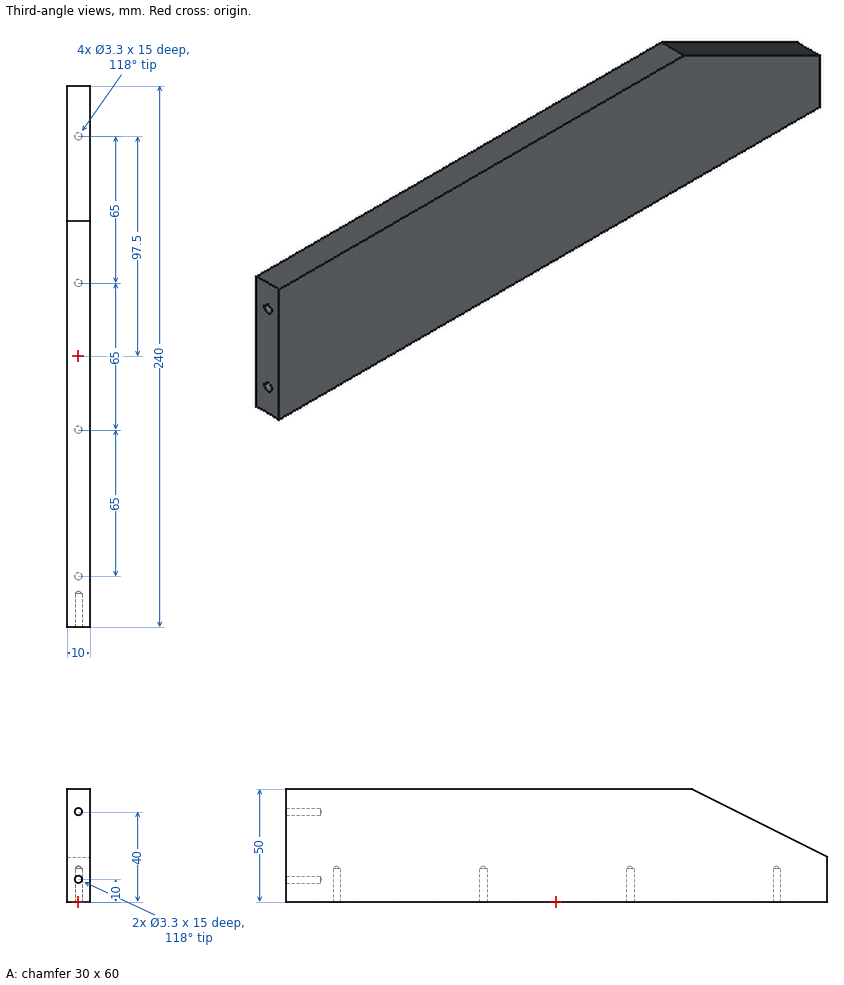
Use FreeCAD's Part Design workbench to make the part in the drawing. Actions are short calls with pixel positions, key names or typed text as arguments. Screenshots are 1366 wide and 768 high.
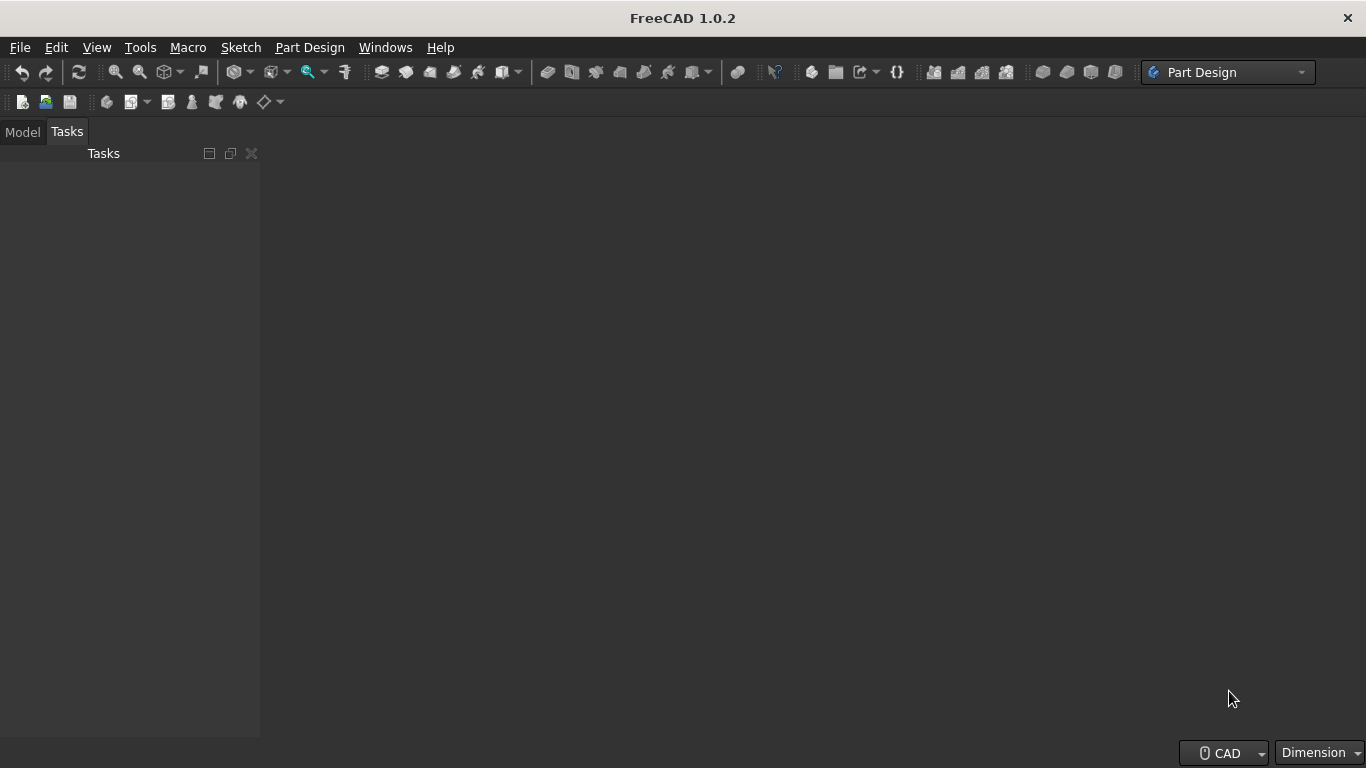
click(22, 102)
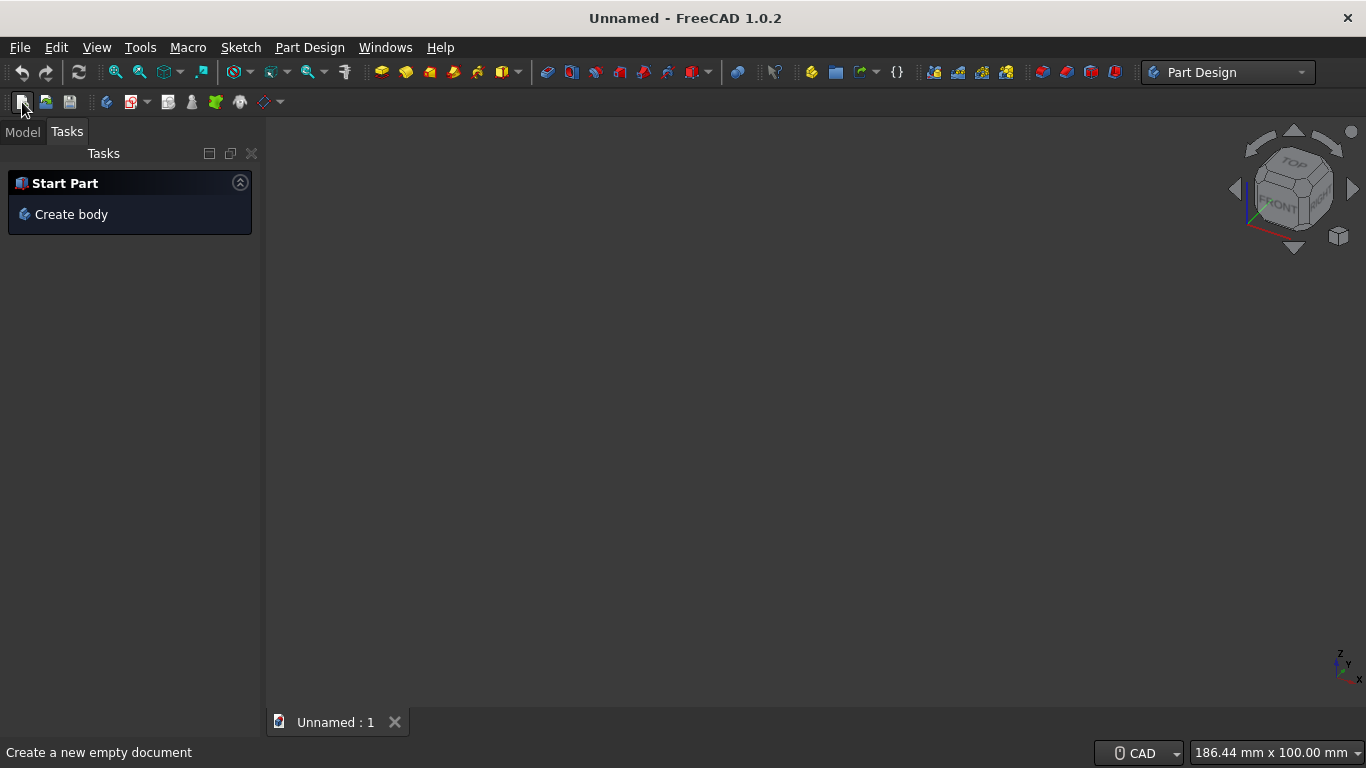
click(132, 102)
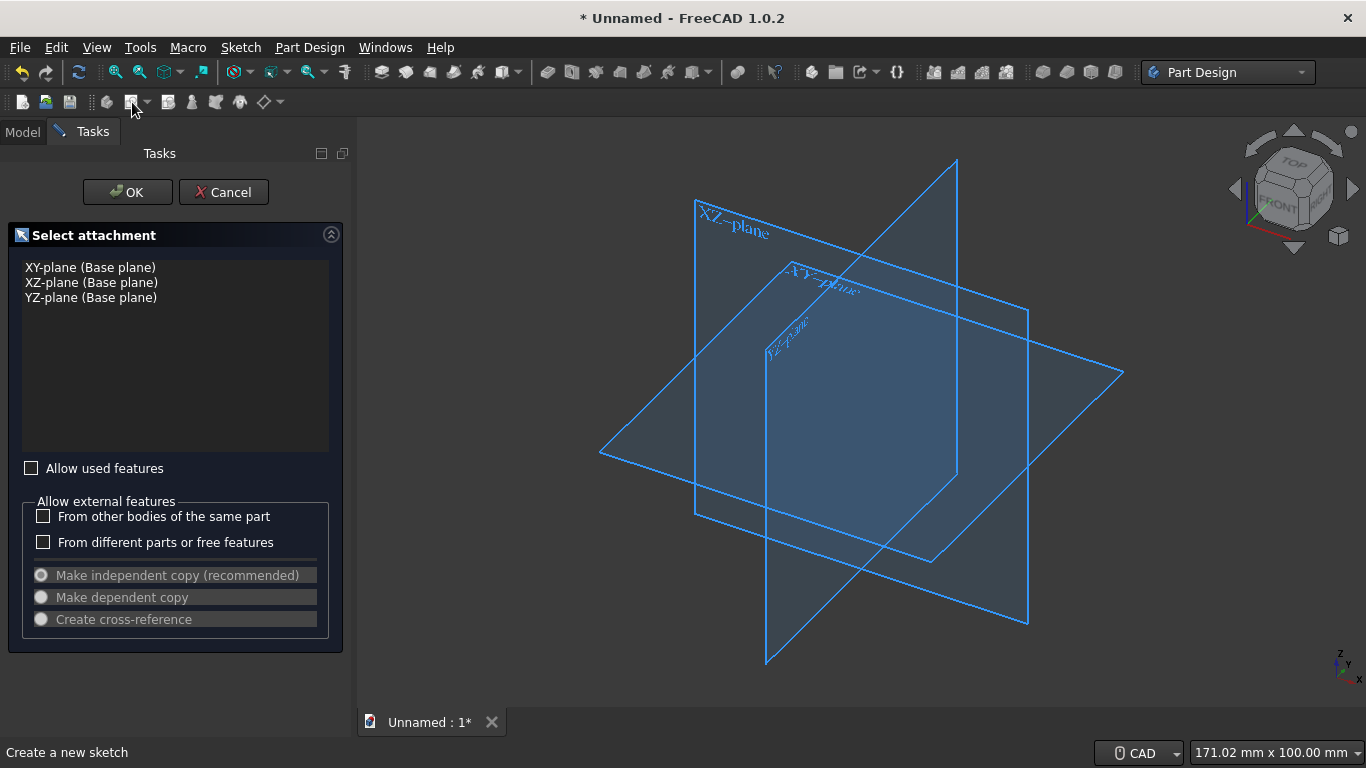
click(82, 268)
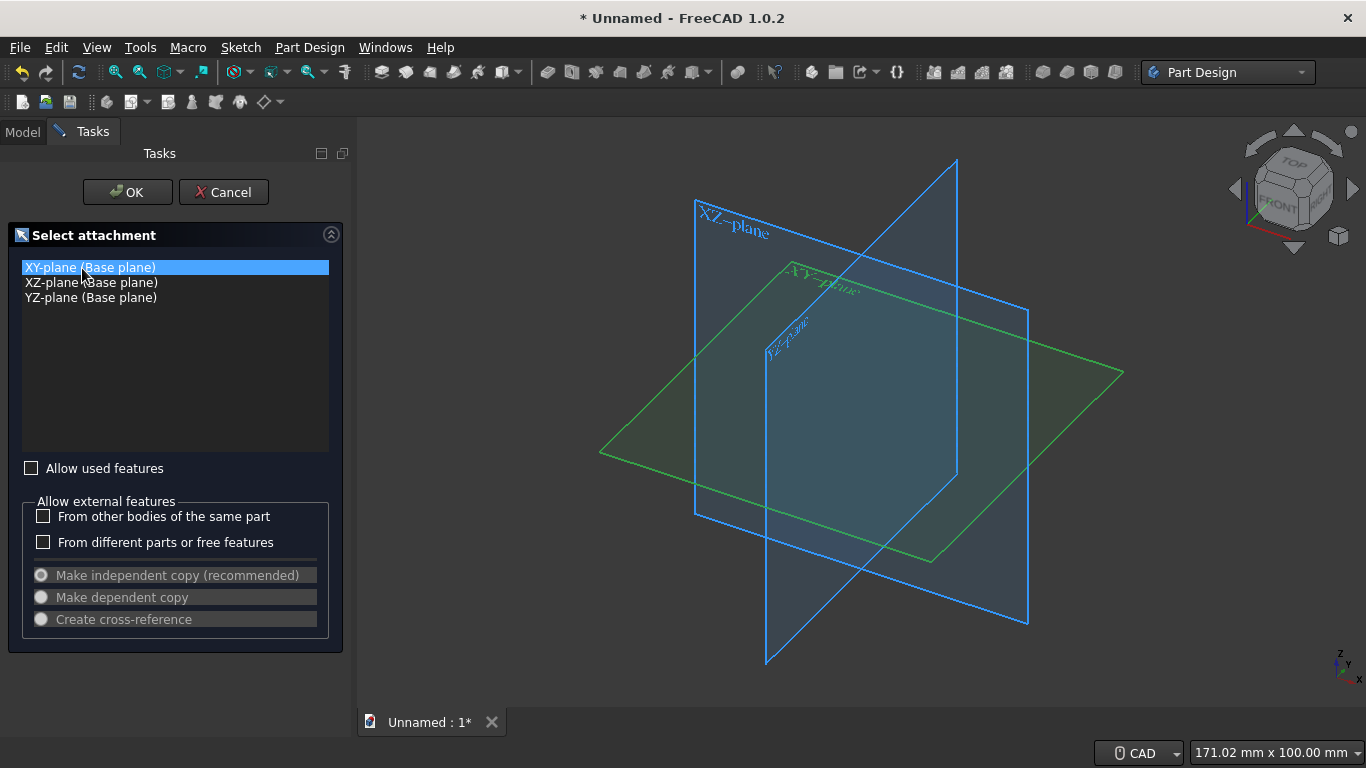
click(128, 192)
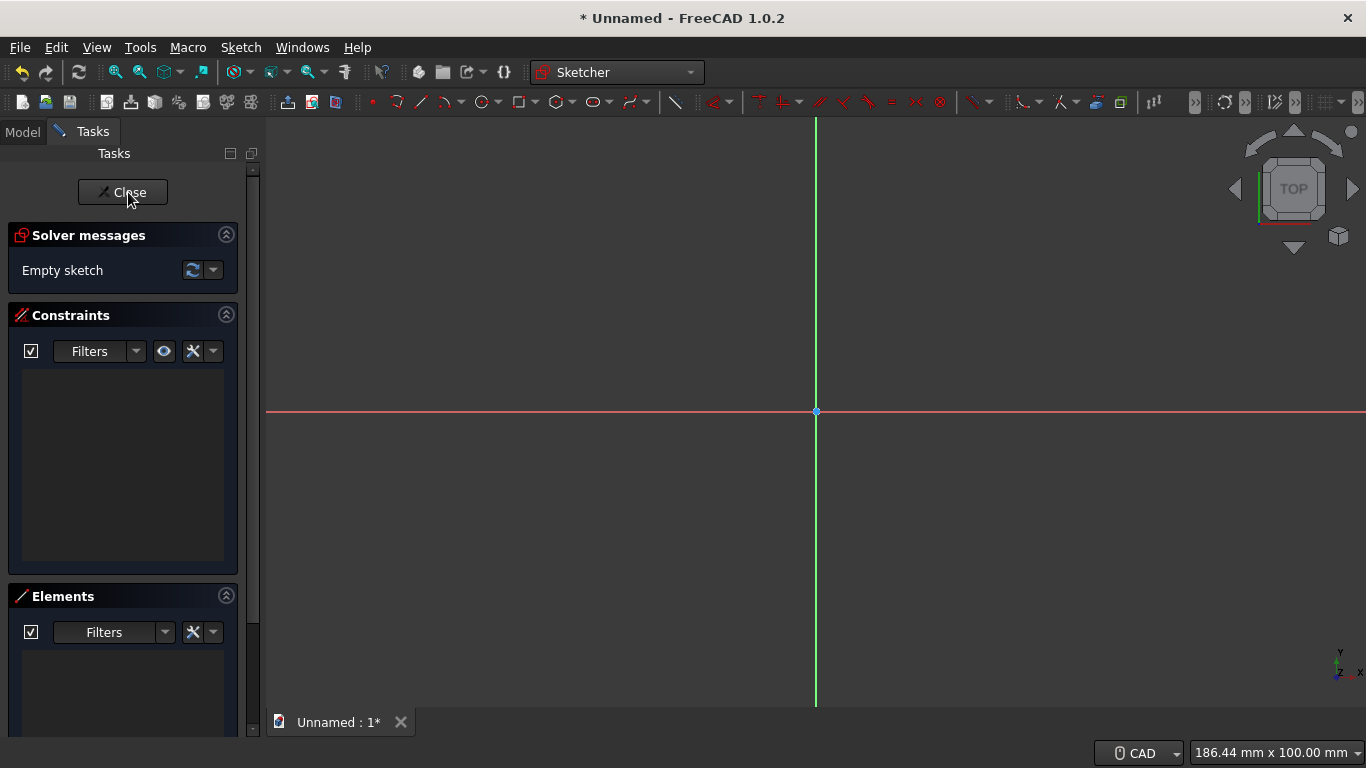
scroll(725, 412, down, 7)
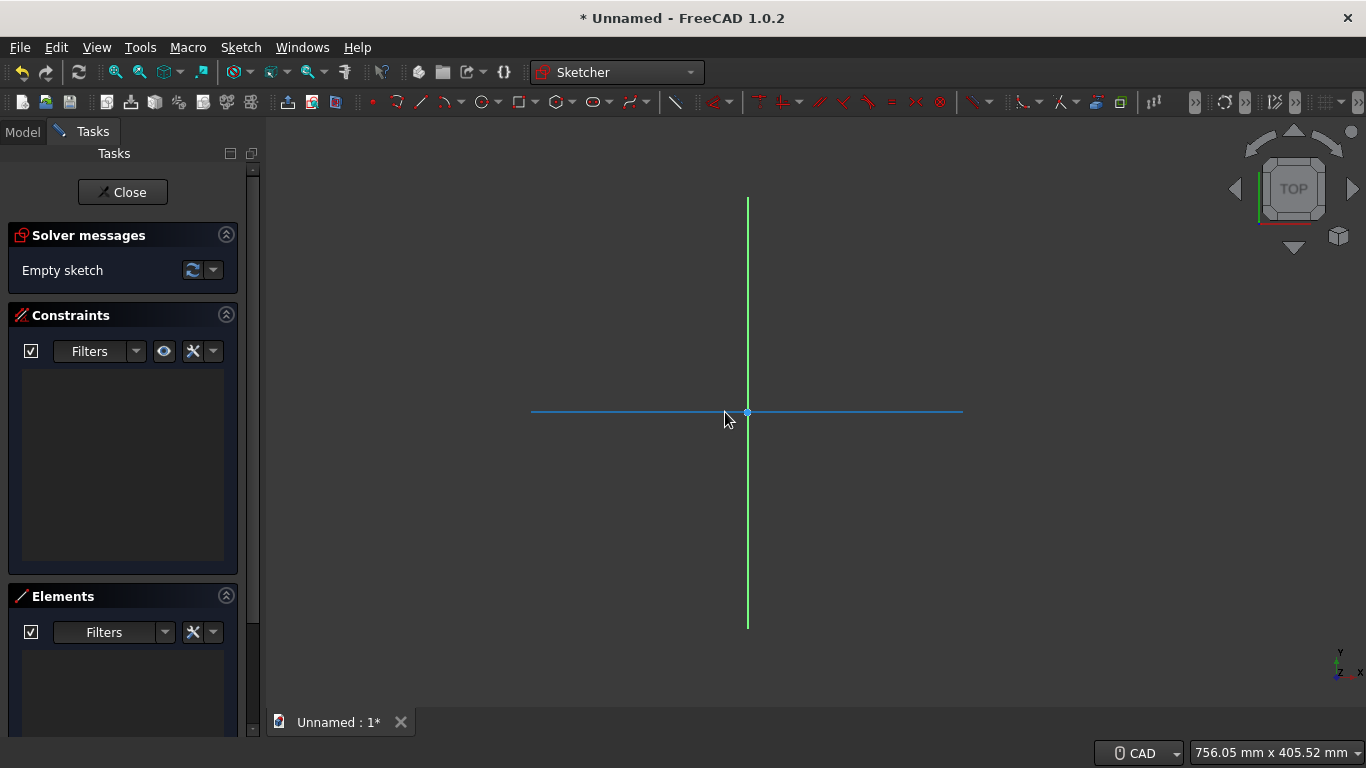
key(g)
key(v)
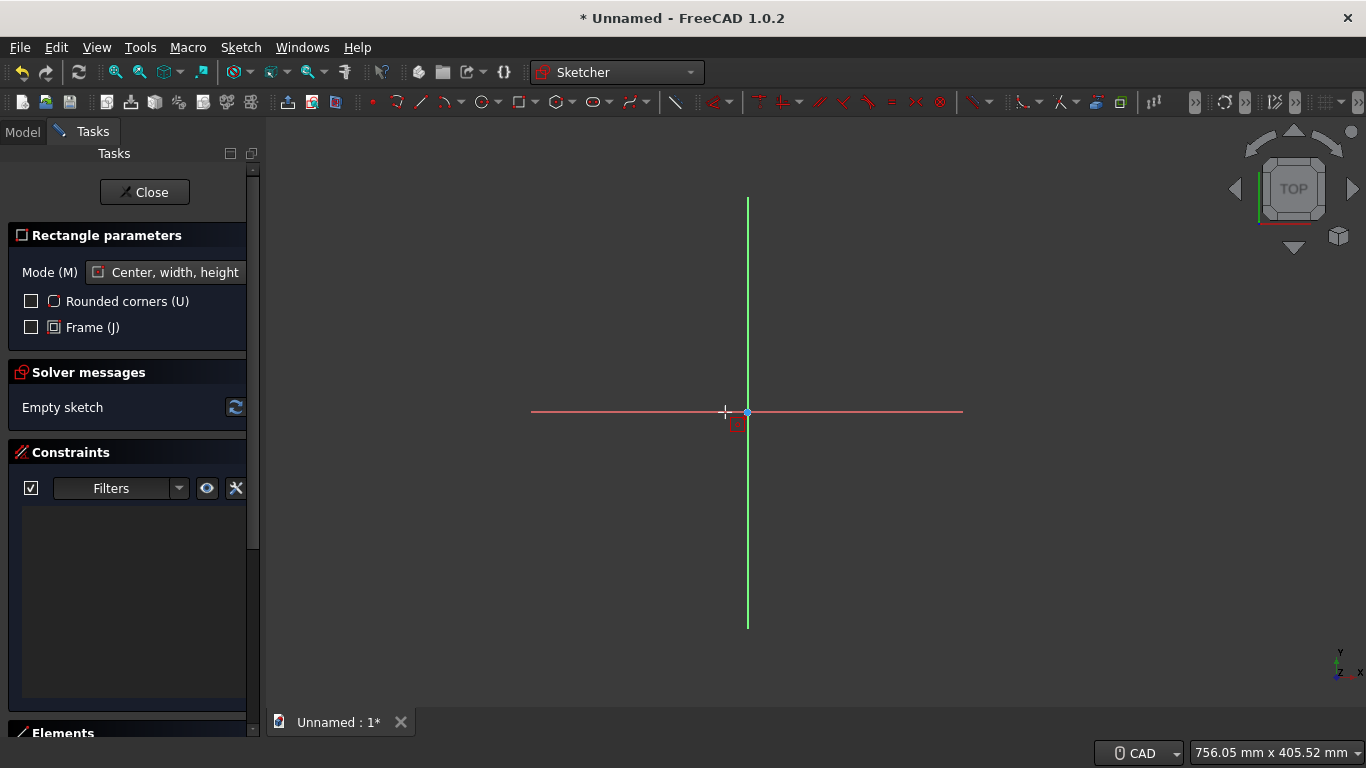
scroll(748, 412, up, 4)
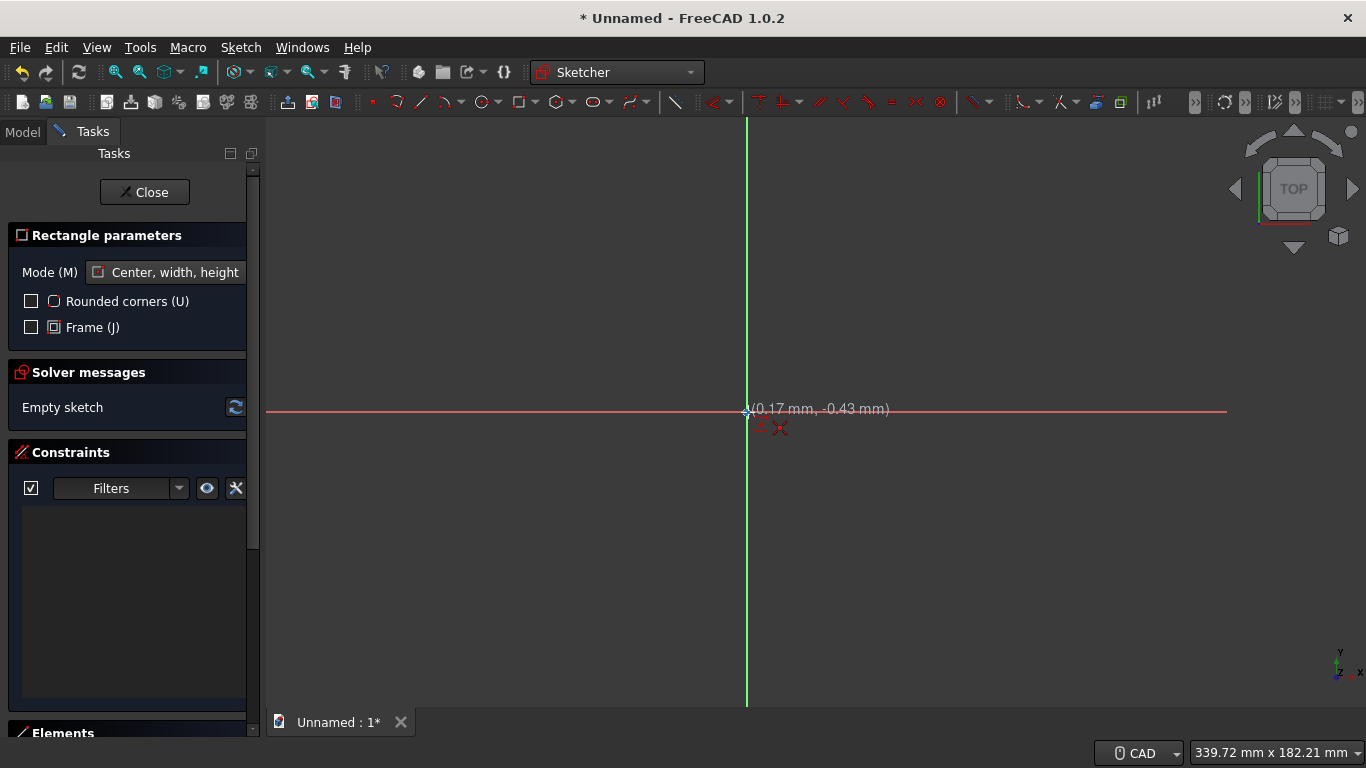
click(747, 412)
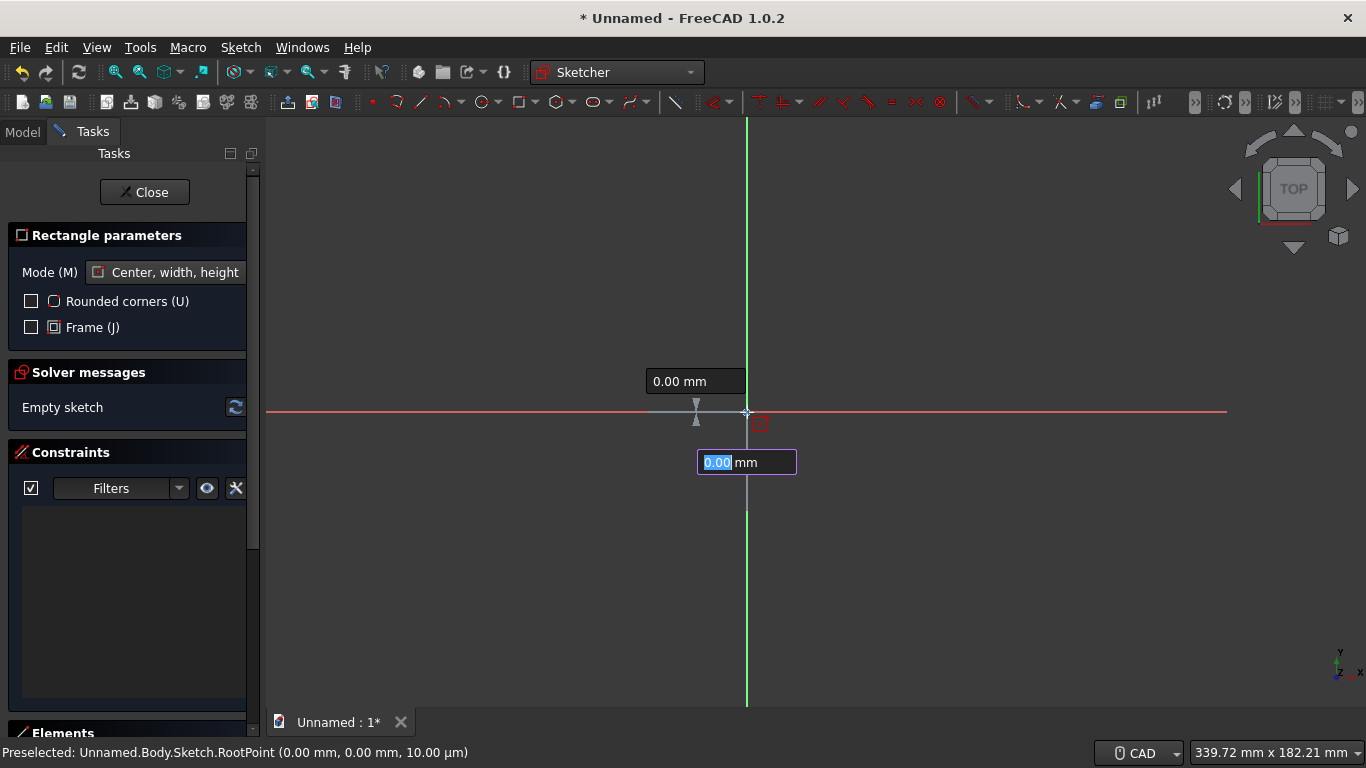
scroll(748, 412, down, 4)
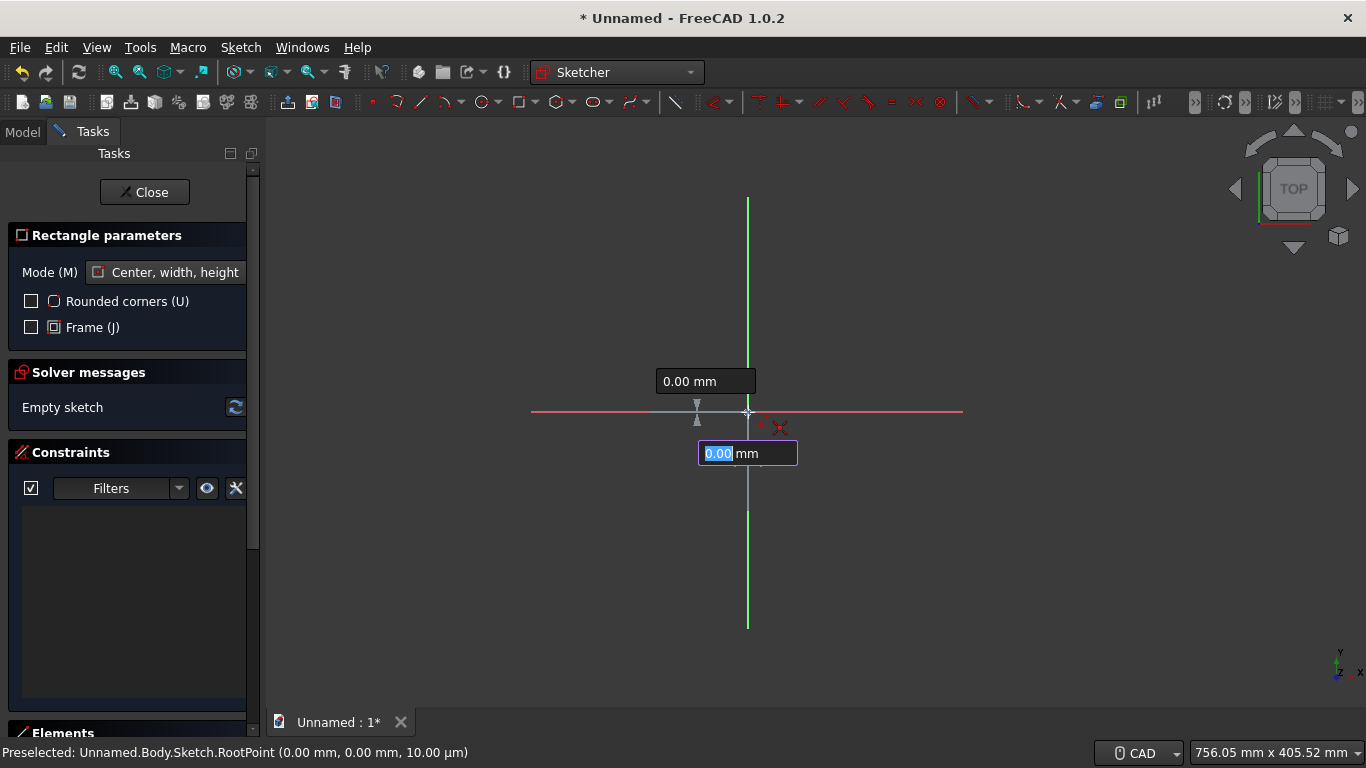
scroll(755, 238, up, 4)